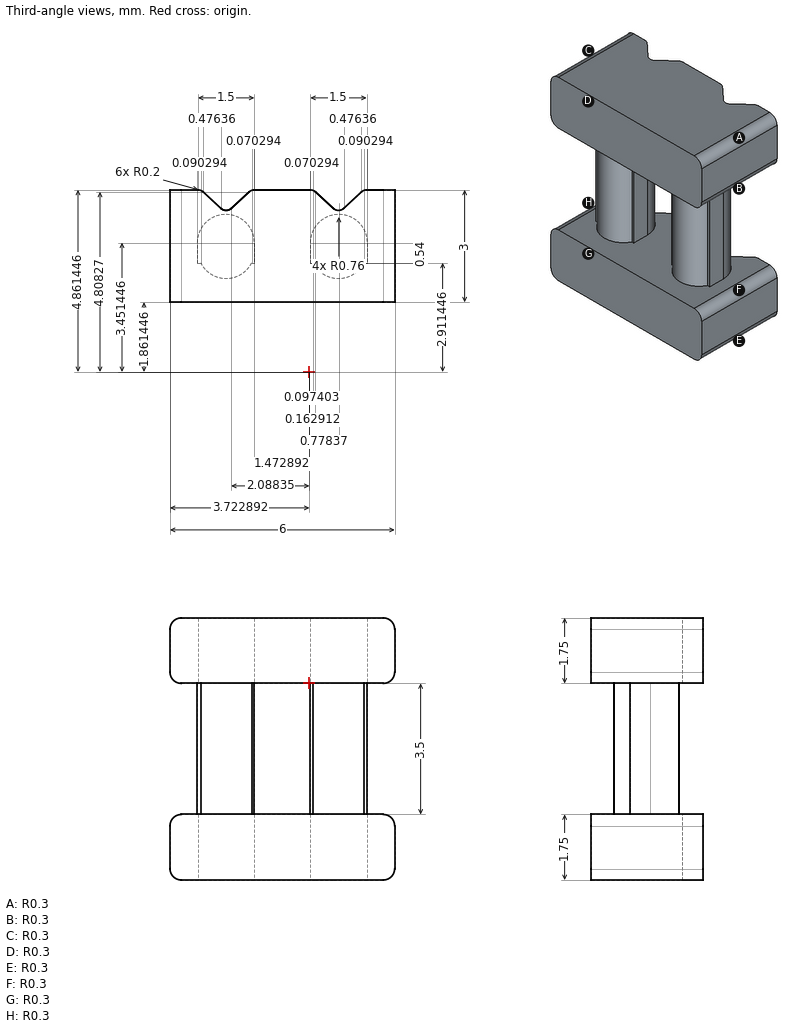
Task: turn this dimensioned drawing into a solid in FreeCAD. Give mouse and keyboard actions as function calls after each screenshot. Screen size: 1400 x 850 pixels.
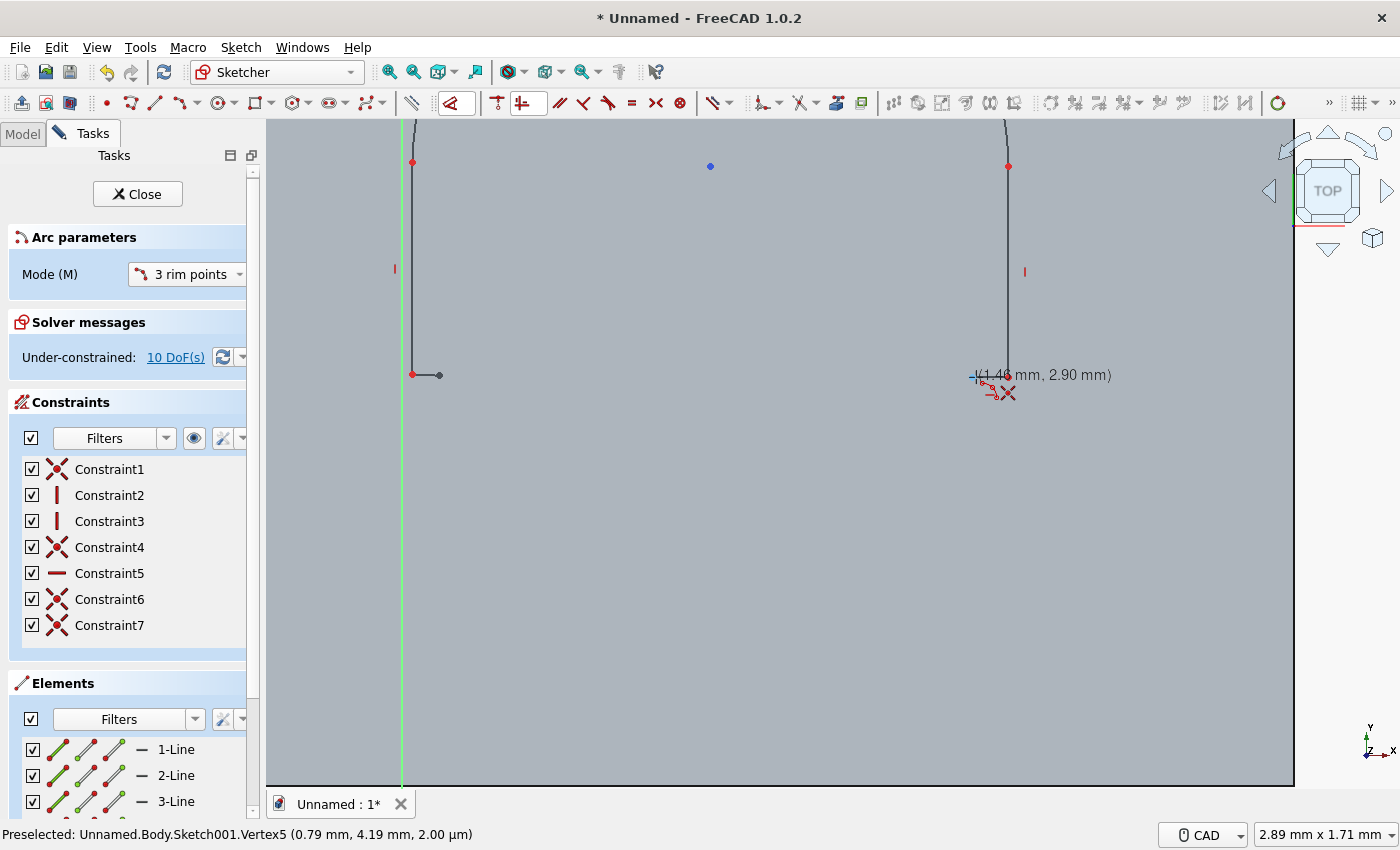
click(973, 377)
click(439, 376)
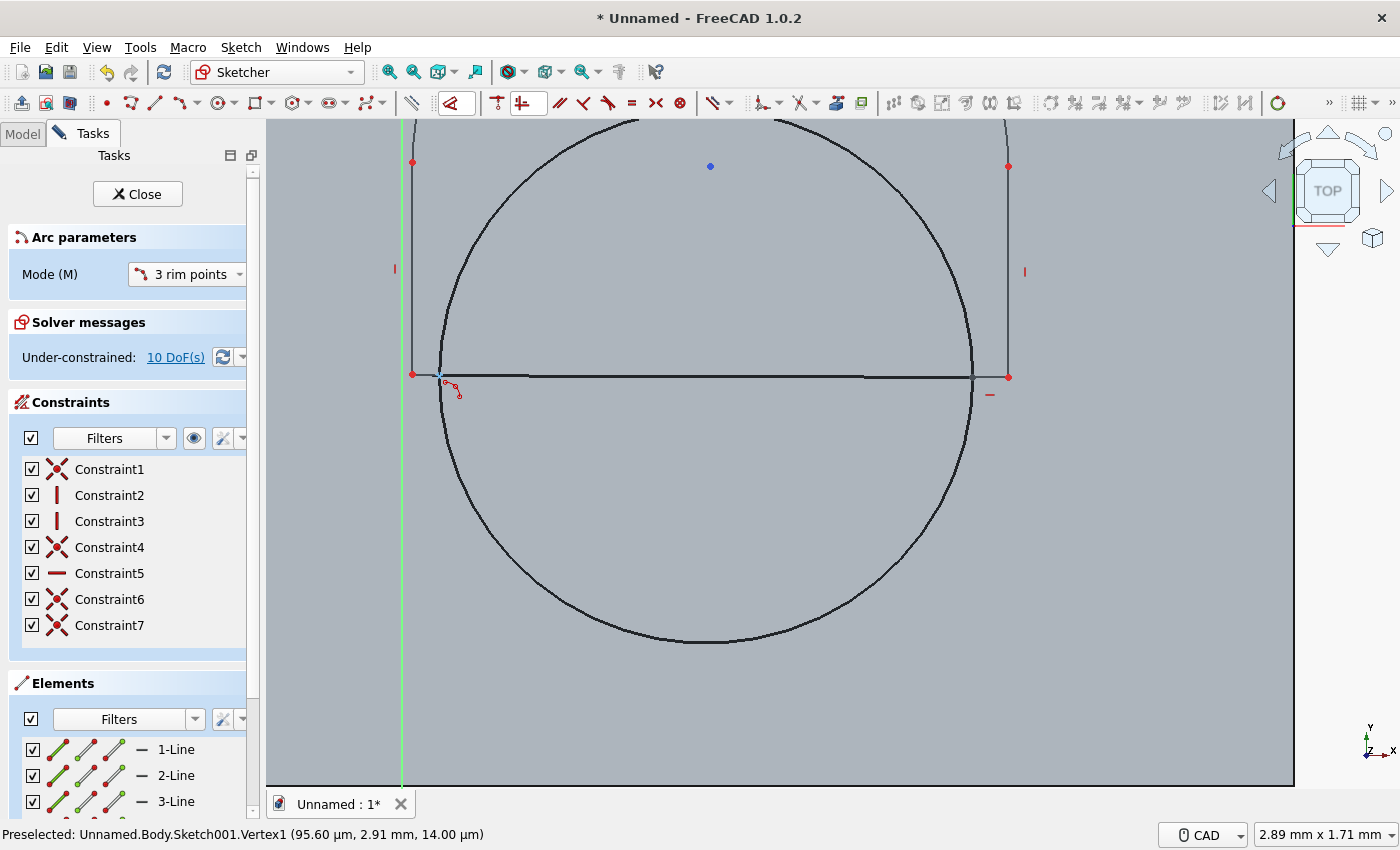
scroll(976, 377, down, 7)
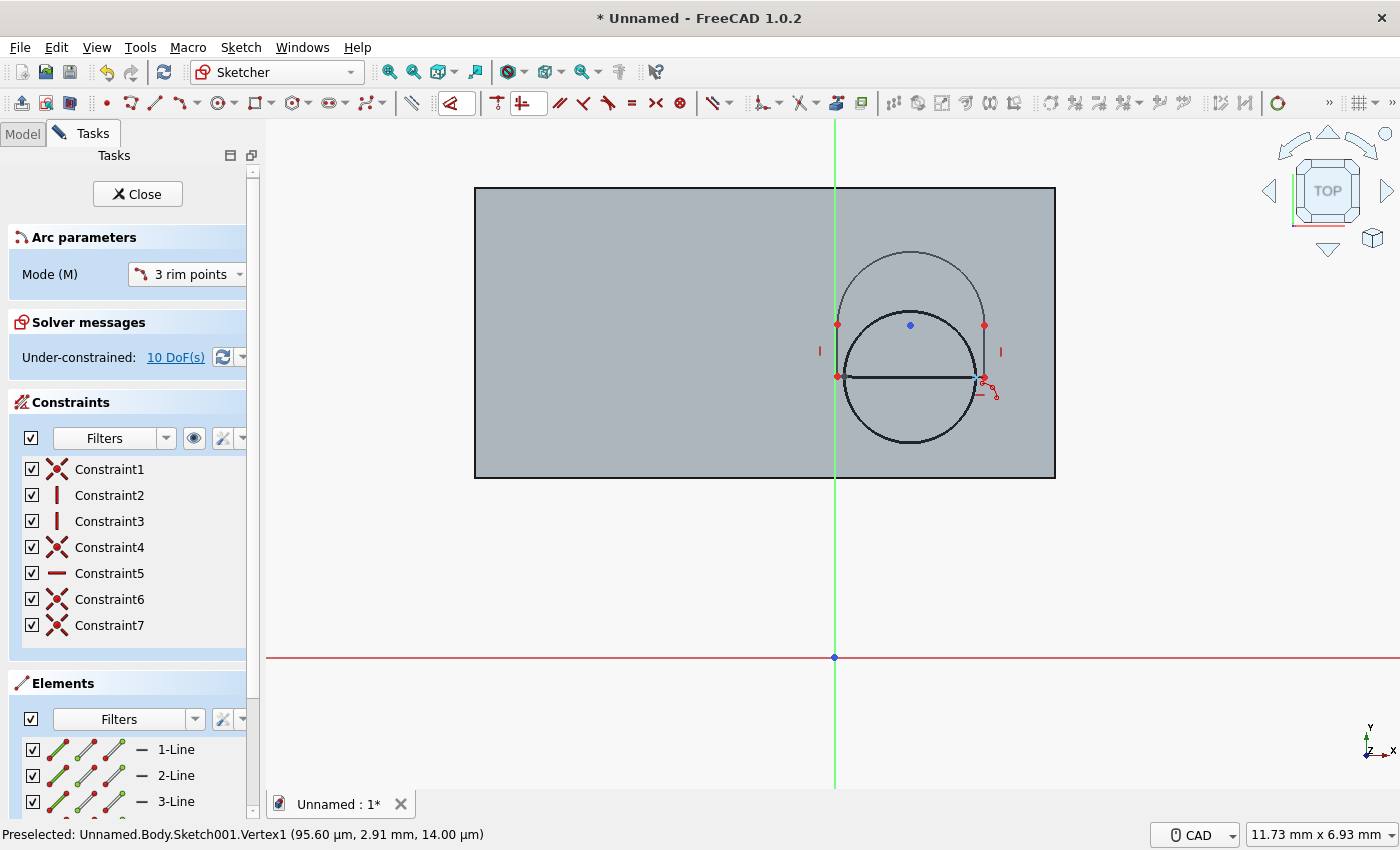
click(910, 417)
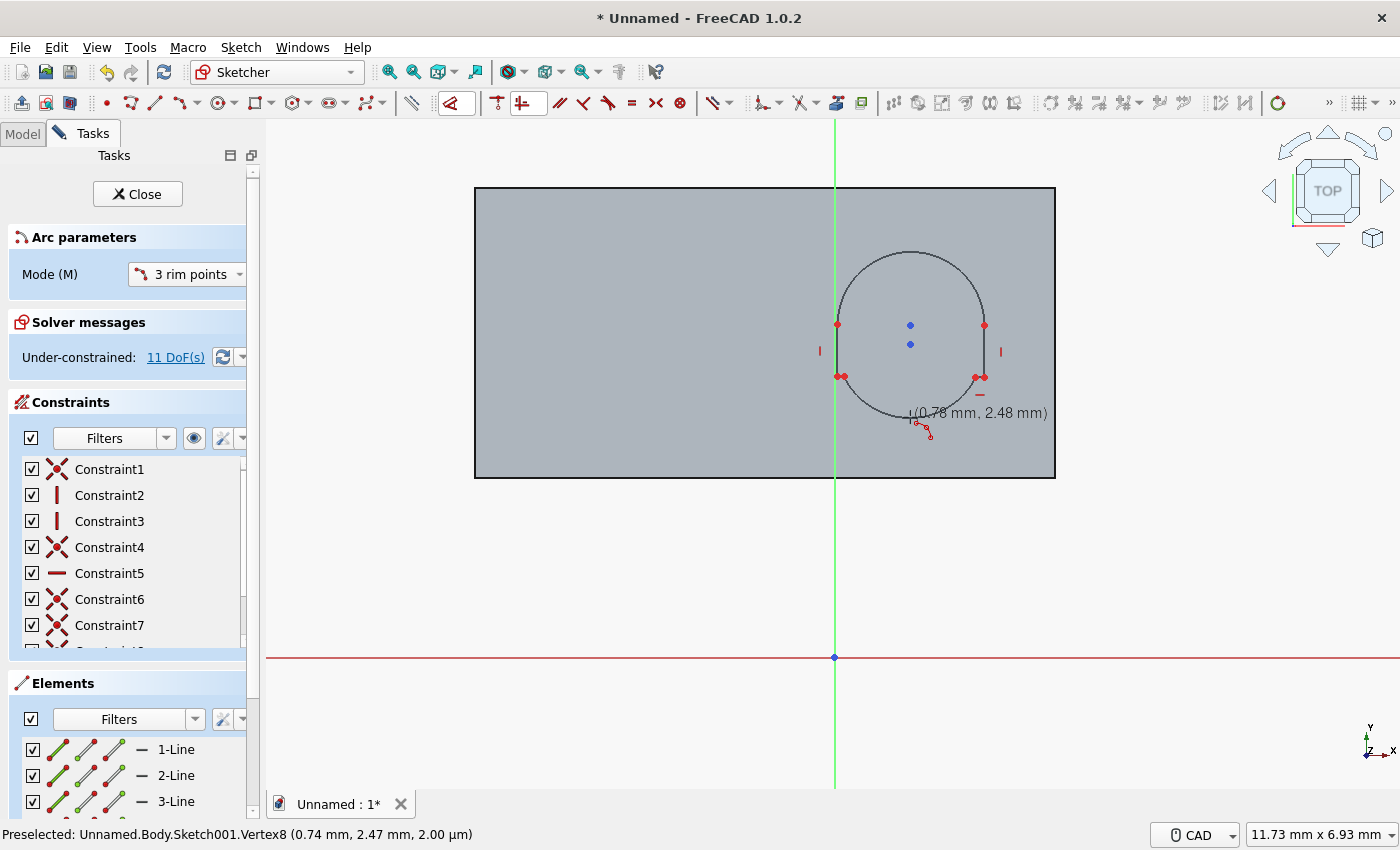
key(g)
key(m)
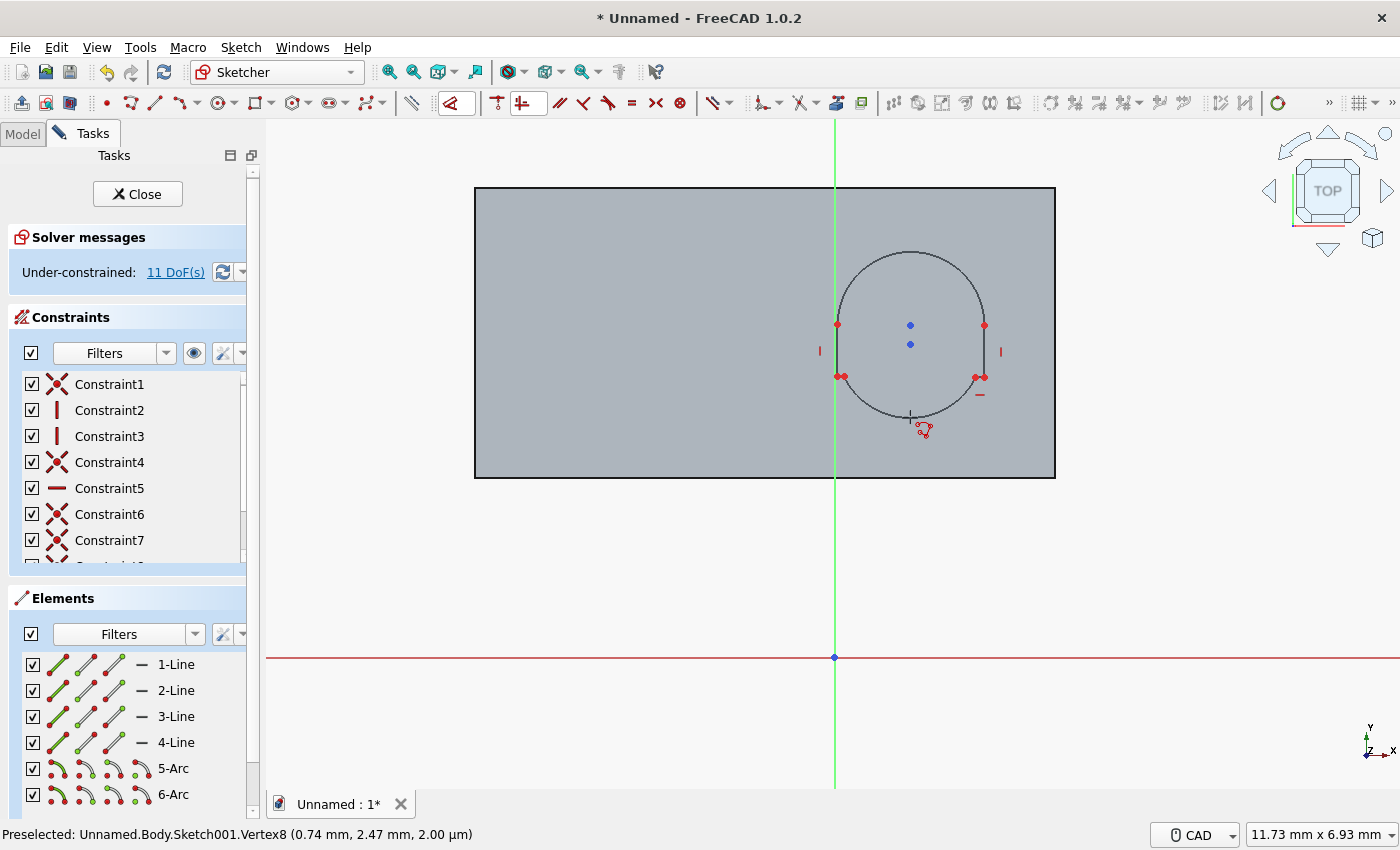
click(693, 324)
click(693, 377)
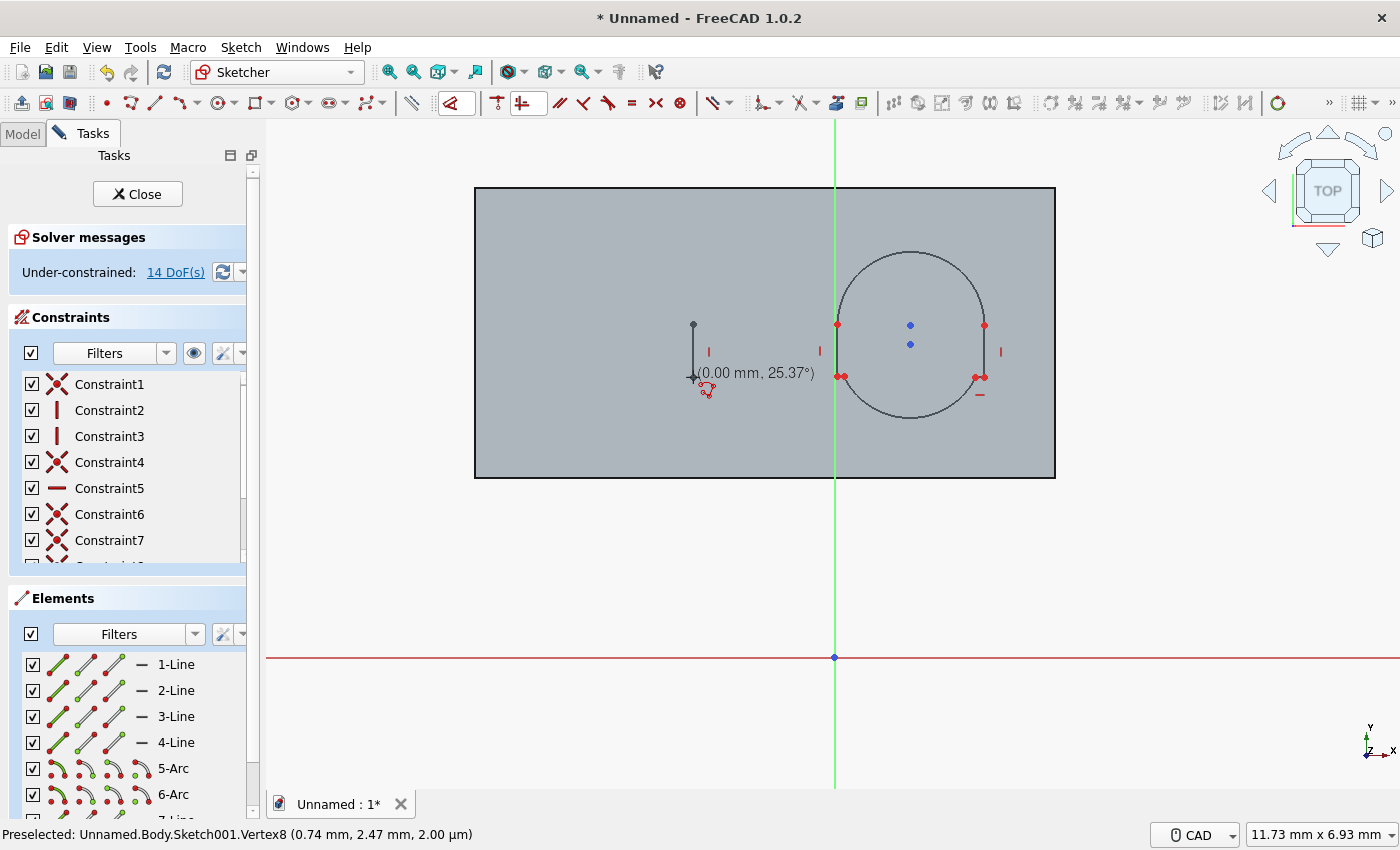
scroll(686, 377, up, 5)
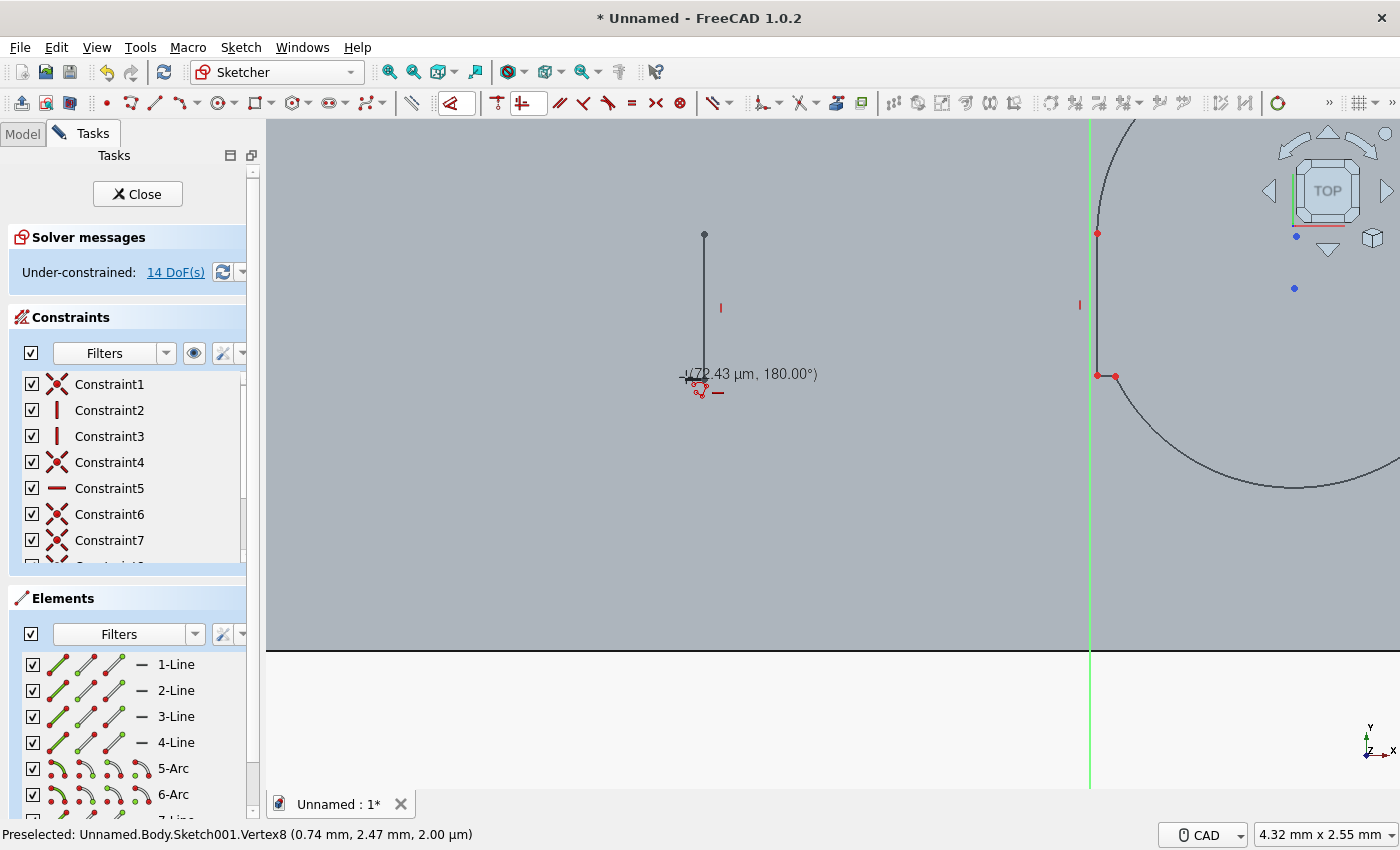
click(685, 376)
right_click(685, 376)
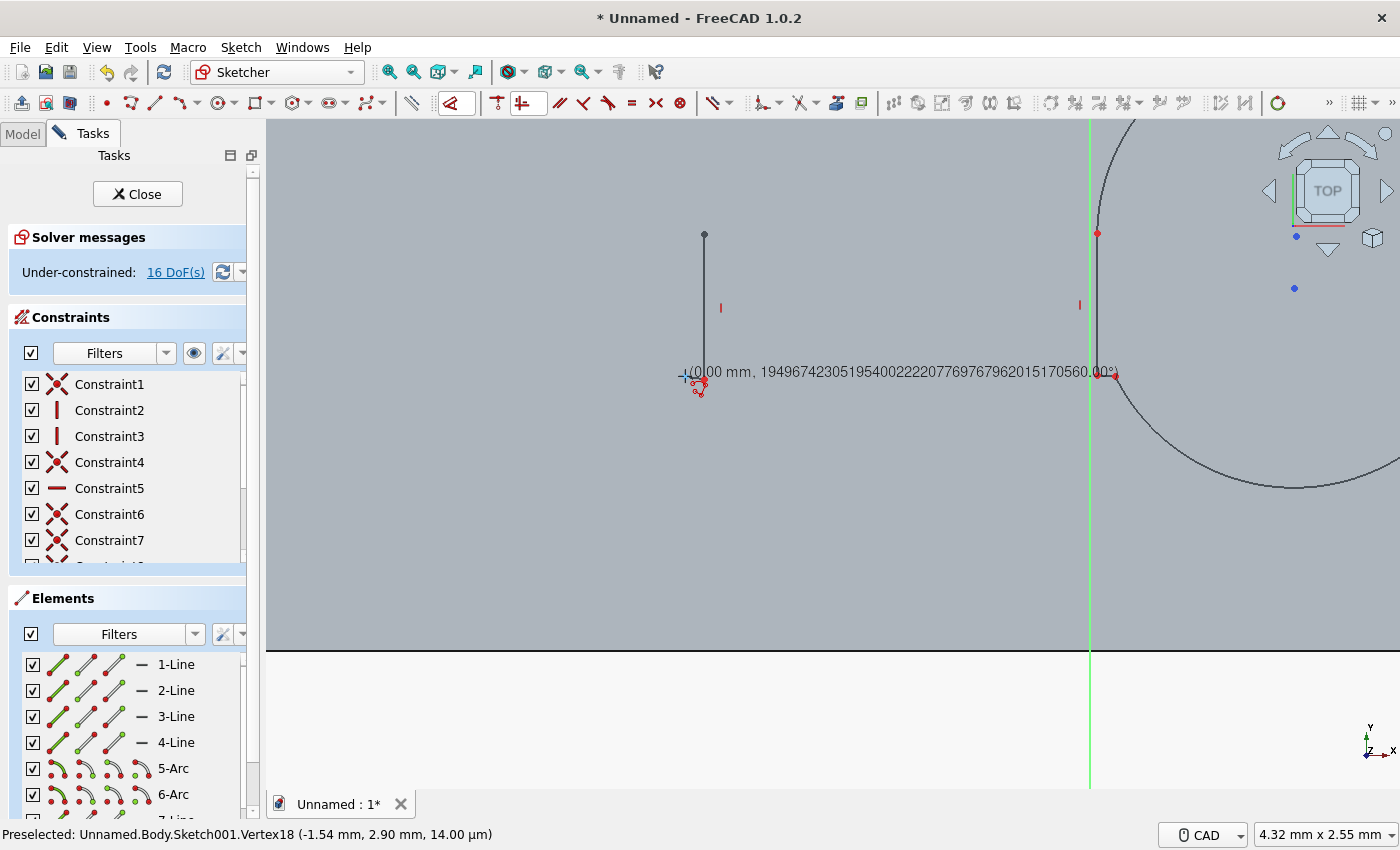
click(328, 375)
click(304, 375)
click(304, 233)
right_click(304, 233)